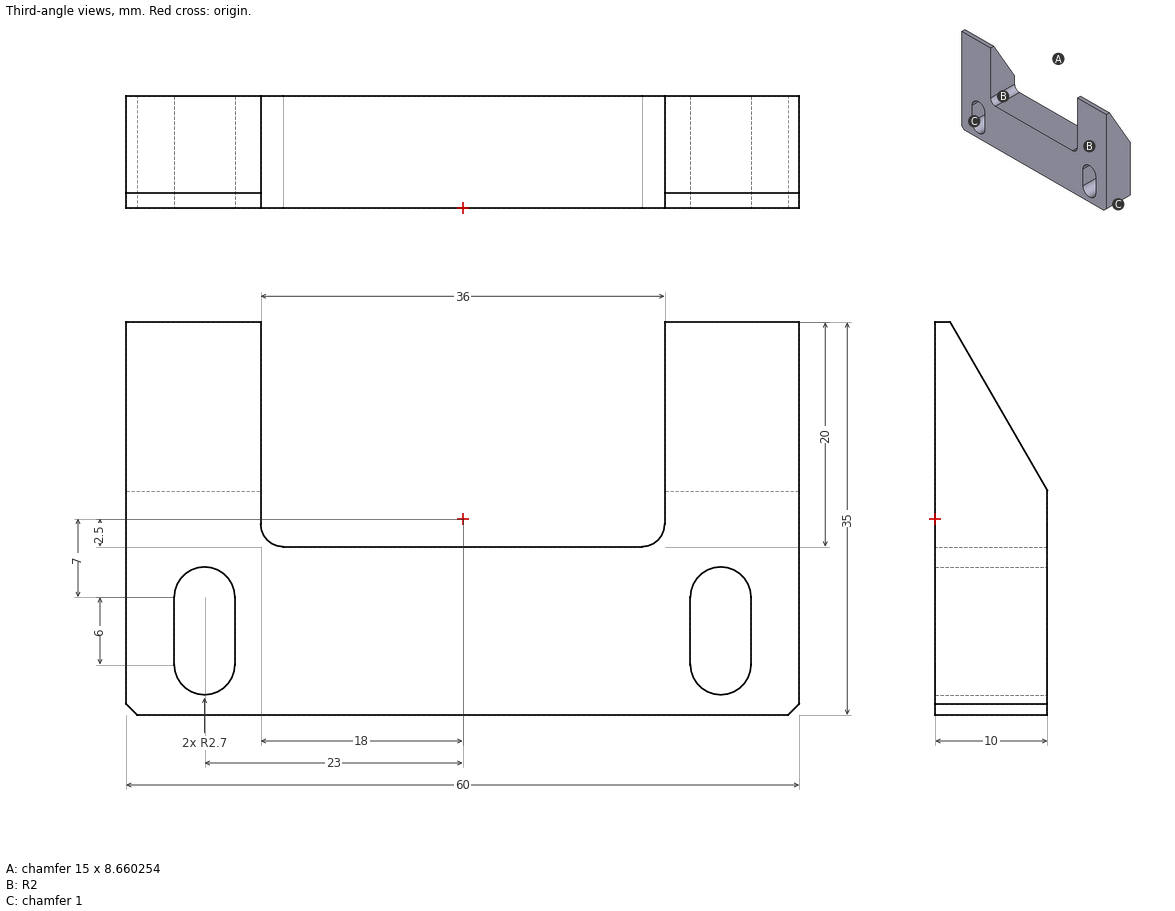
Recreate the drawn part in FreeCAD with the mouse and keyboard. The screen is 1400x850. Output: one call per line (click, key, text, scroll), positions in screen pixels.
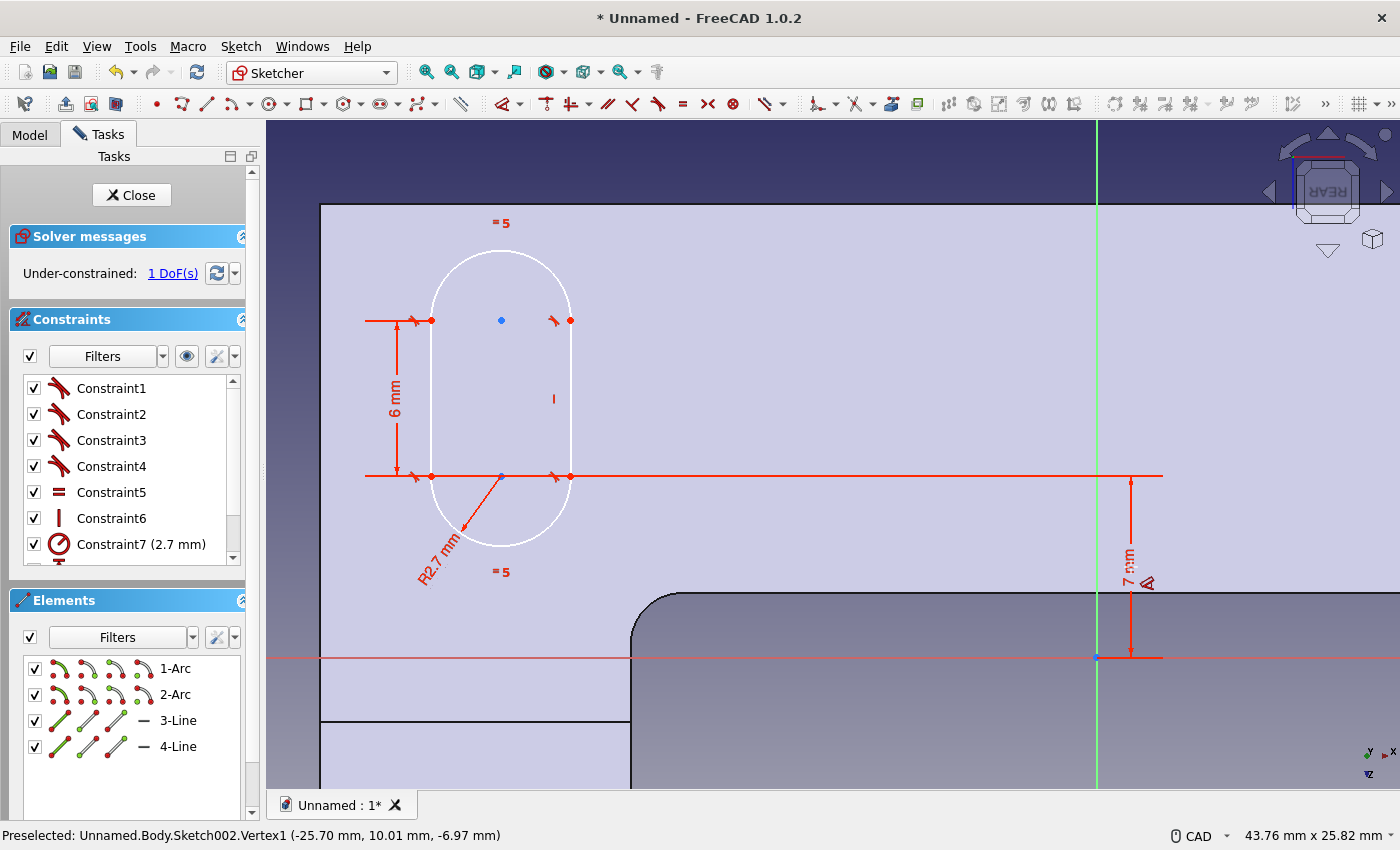
click(501, 476)
click(799, 692)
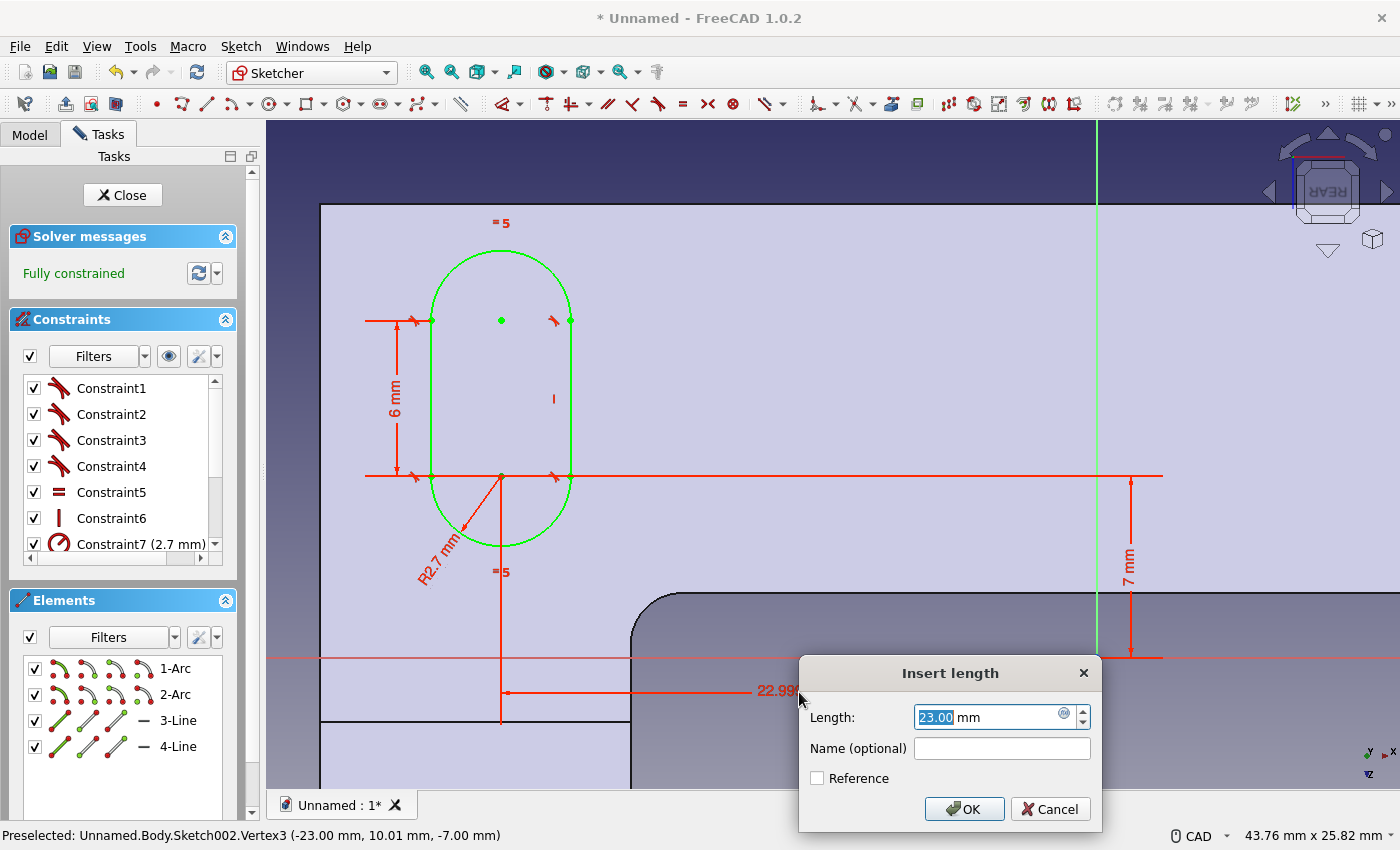
text(23)
key(Return)
key(Escape)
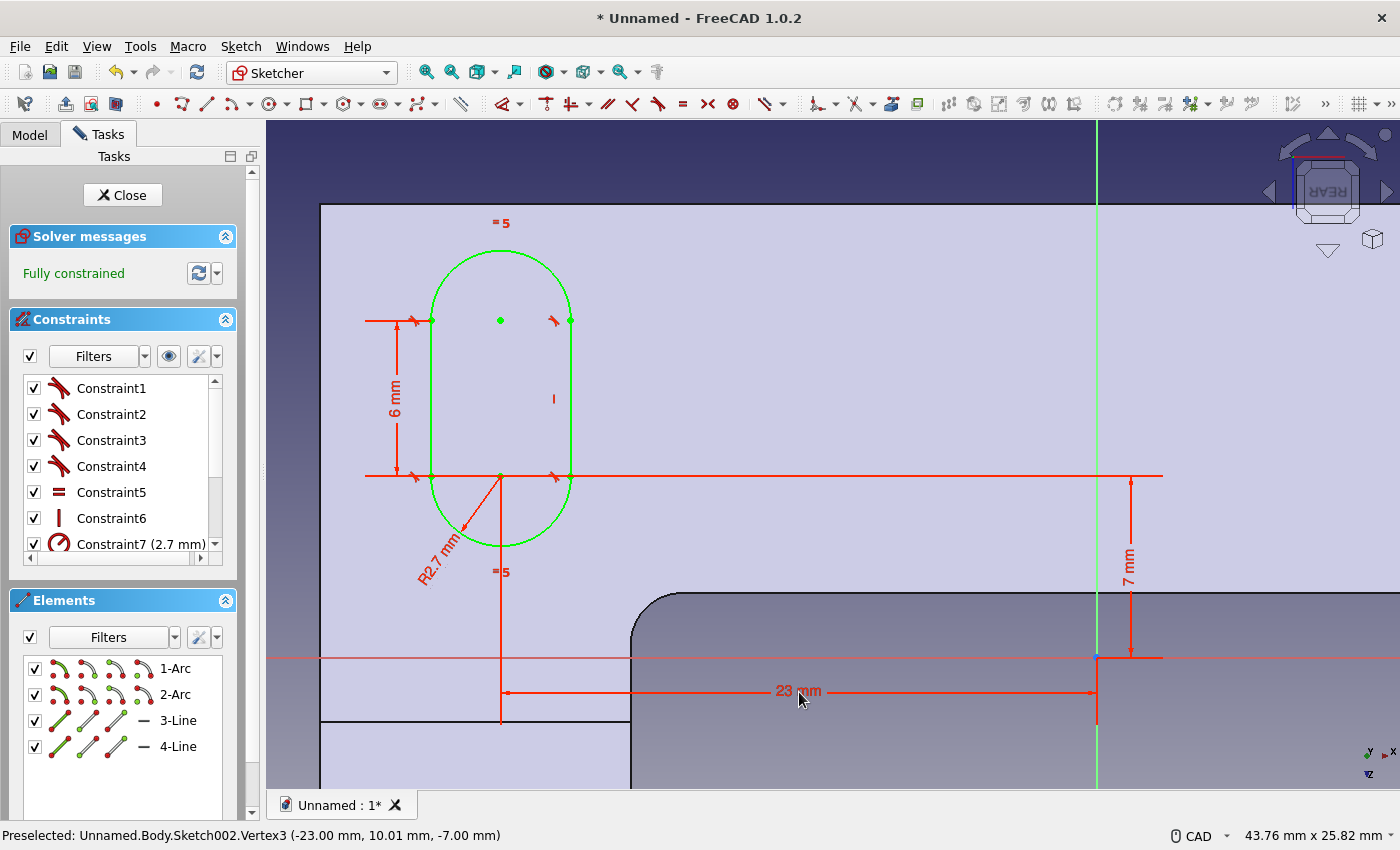
click(123, 195)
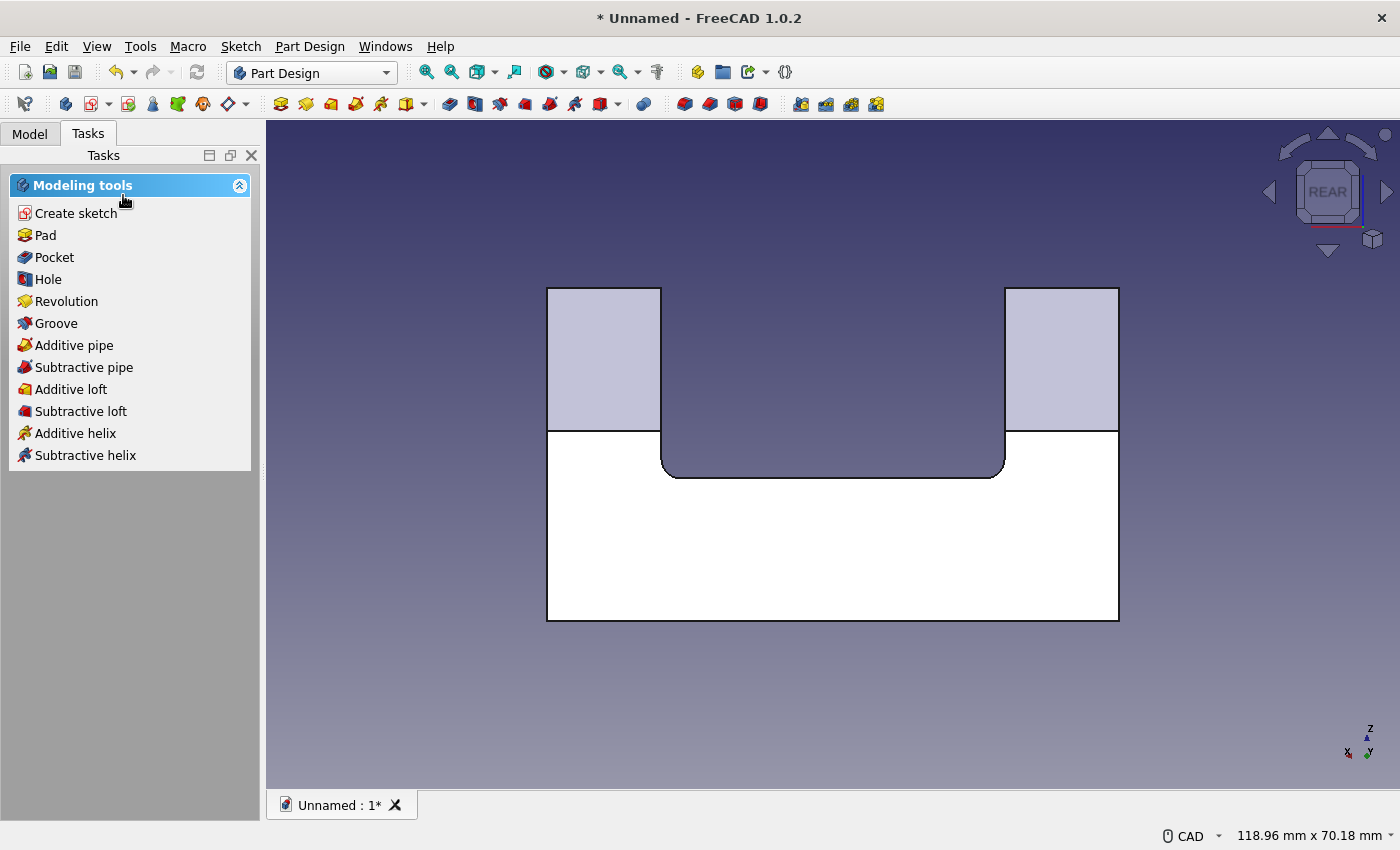
click(450, 104)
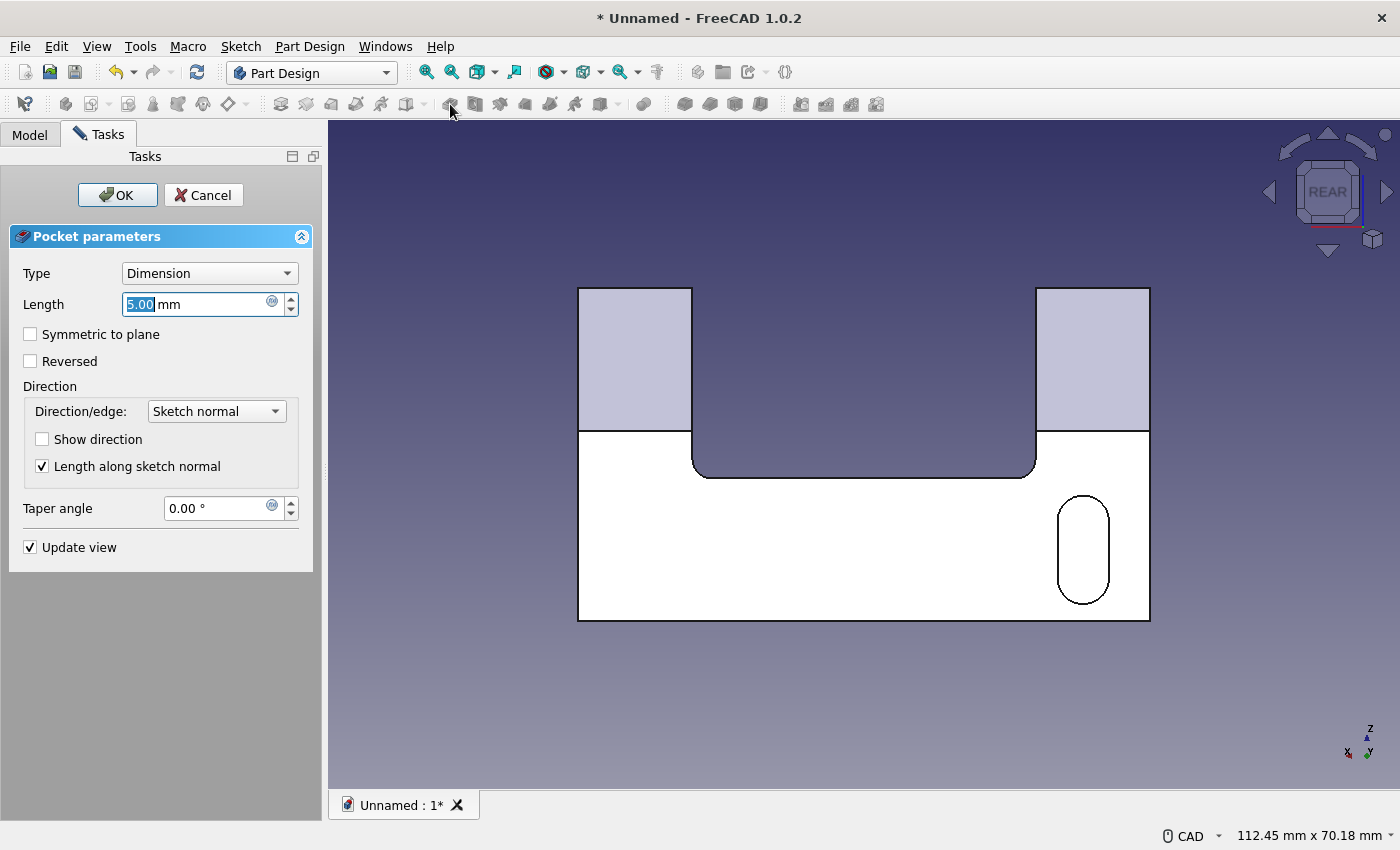
click(210, 274)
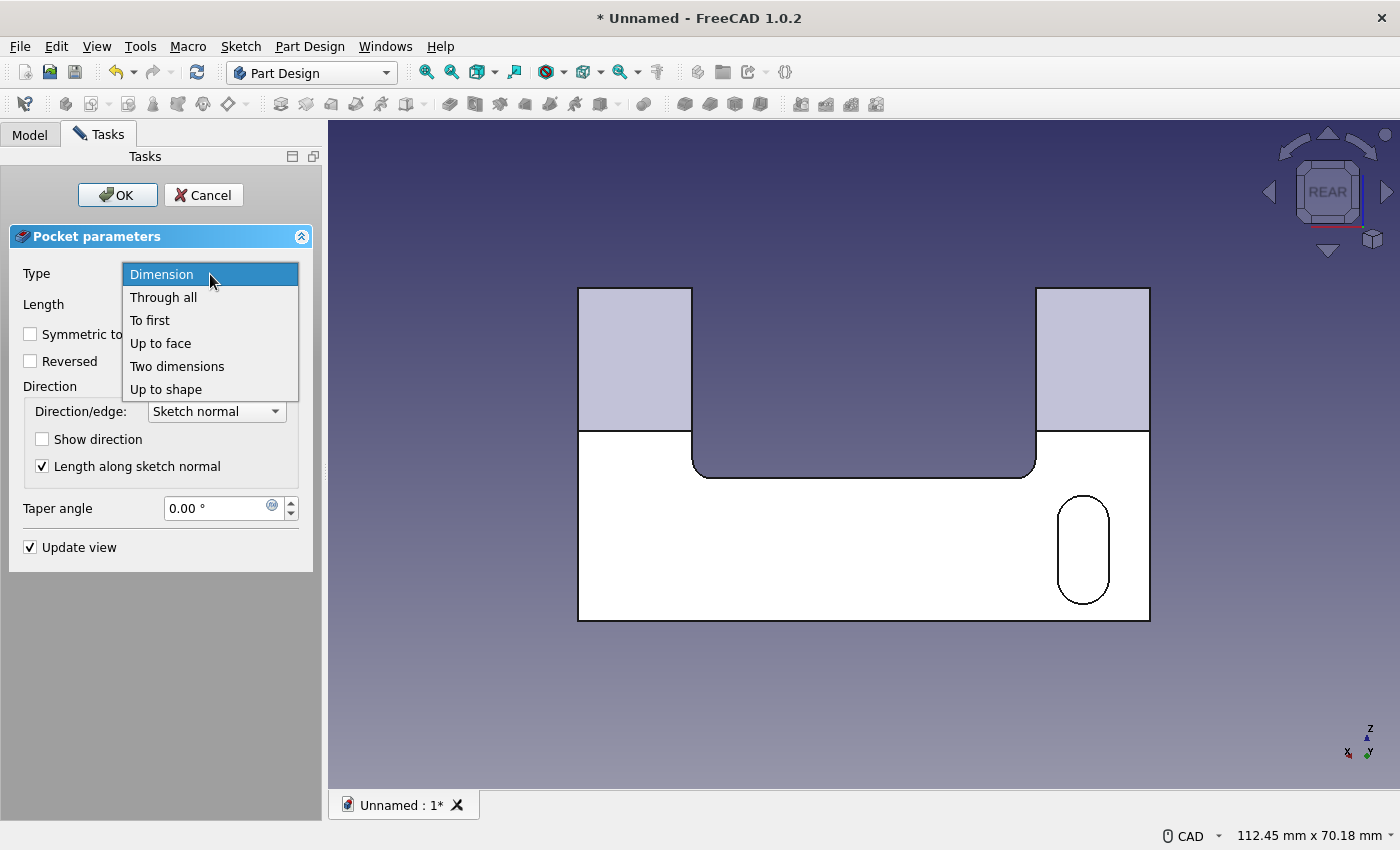
click(208, 298)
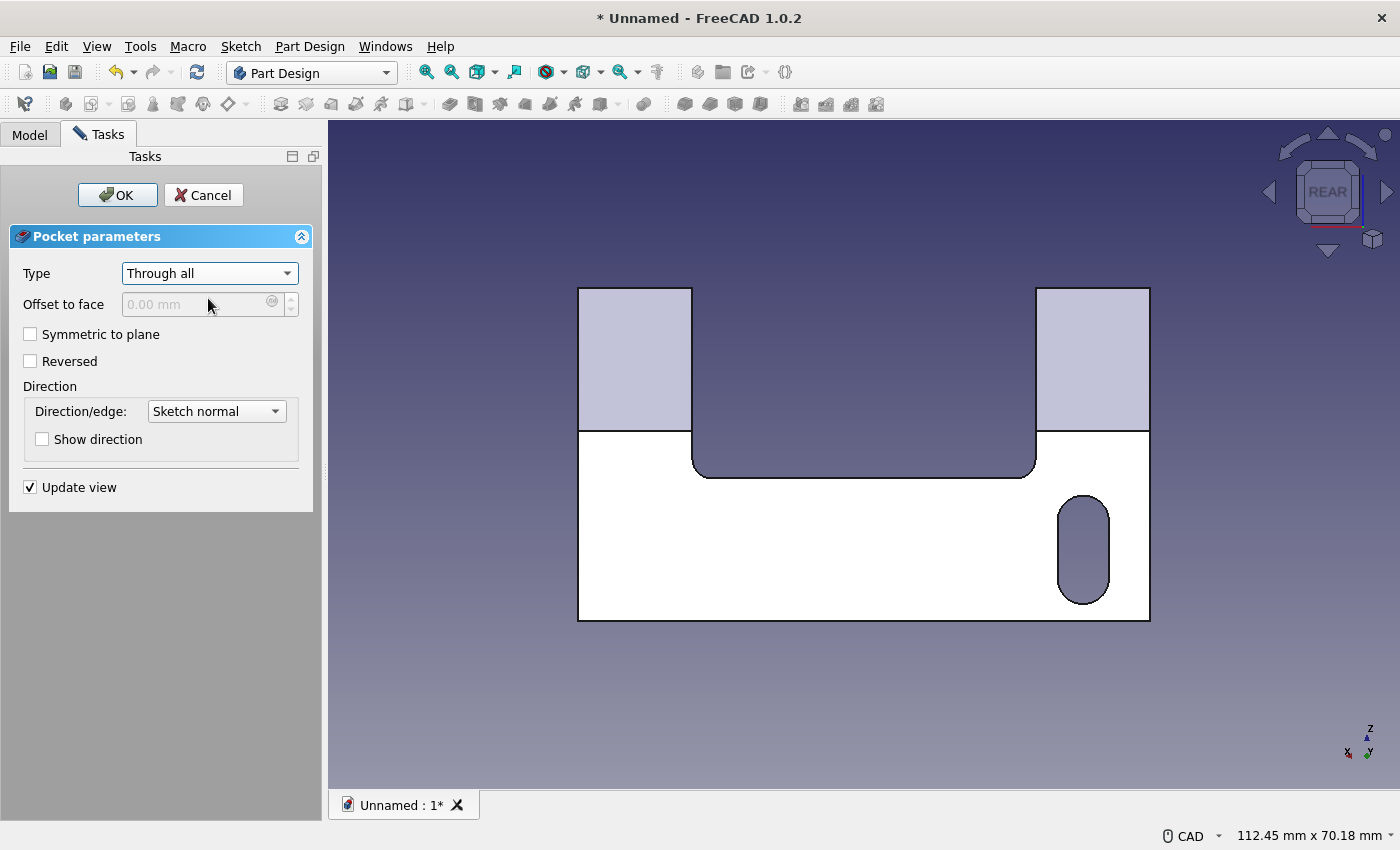
click(118, 195)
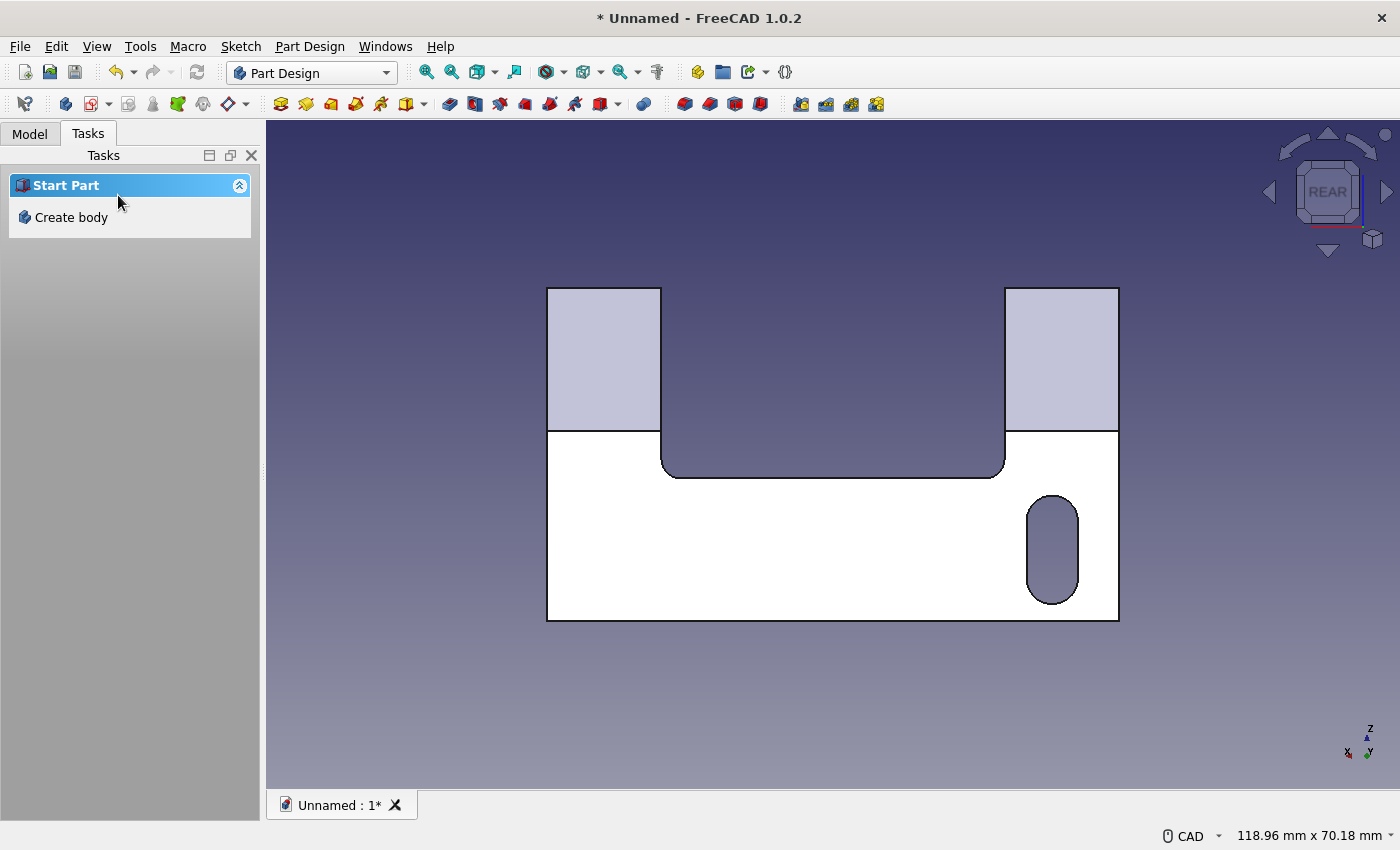
click(30, 134)